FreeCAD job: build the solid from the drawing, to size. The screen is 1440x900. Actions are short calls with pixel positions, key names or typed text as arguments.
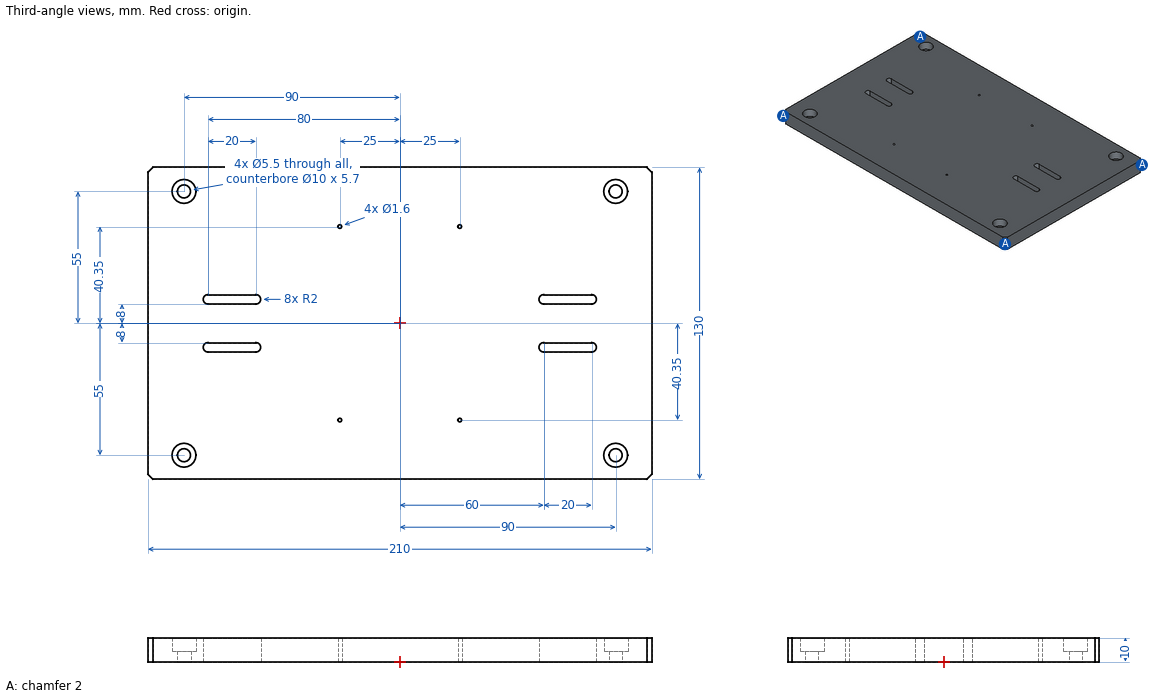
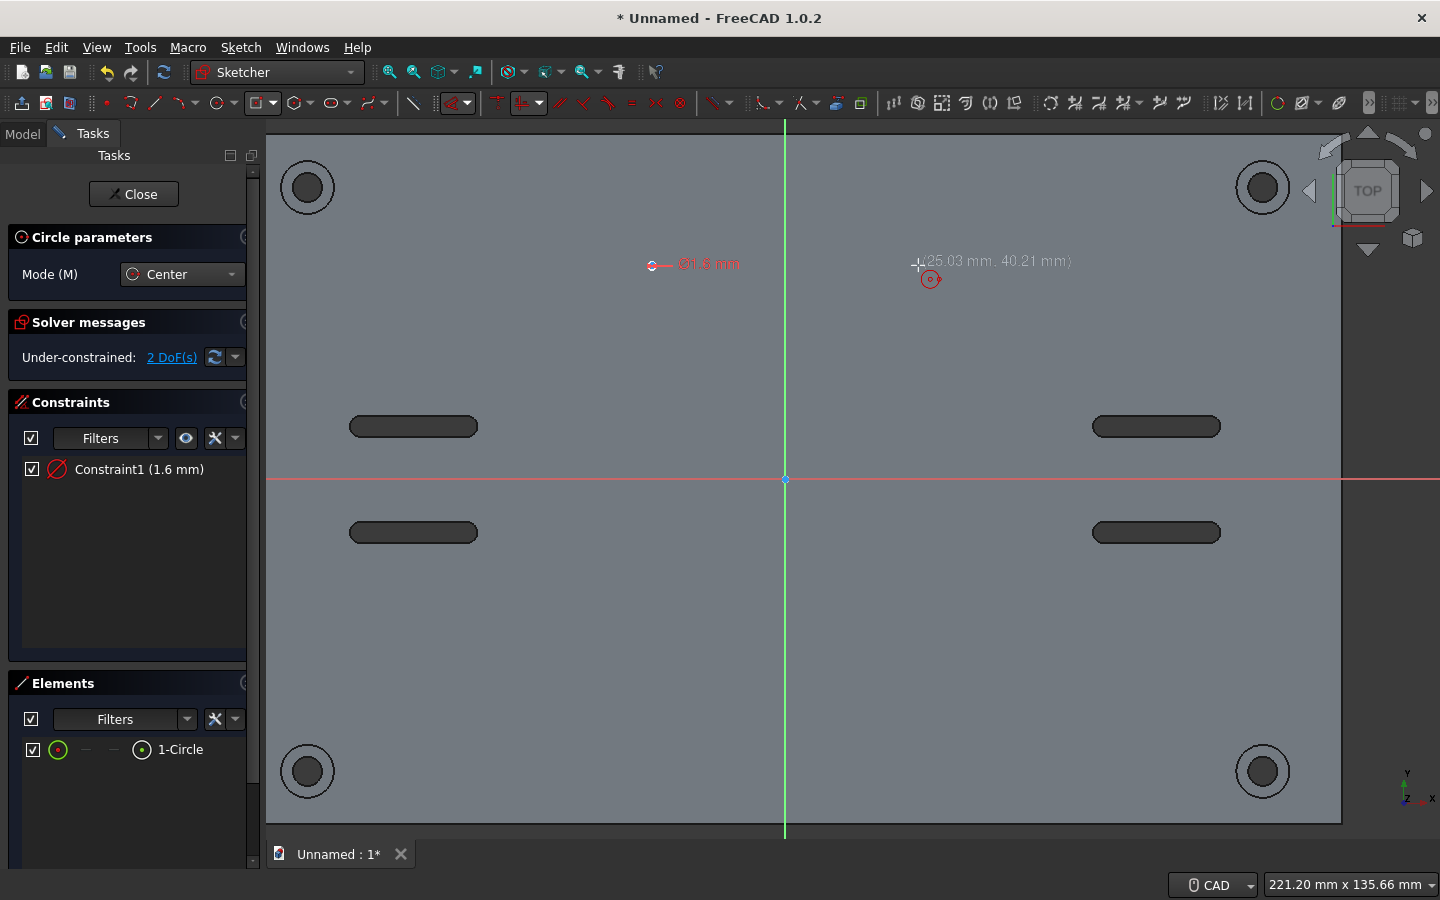
click(918, 265)
move(921, 262)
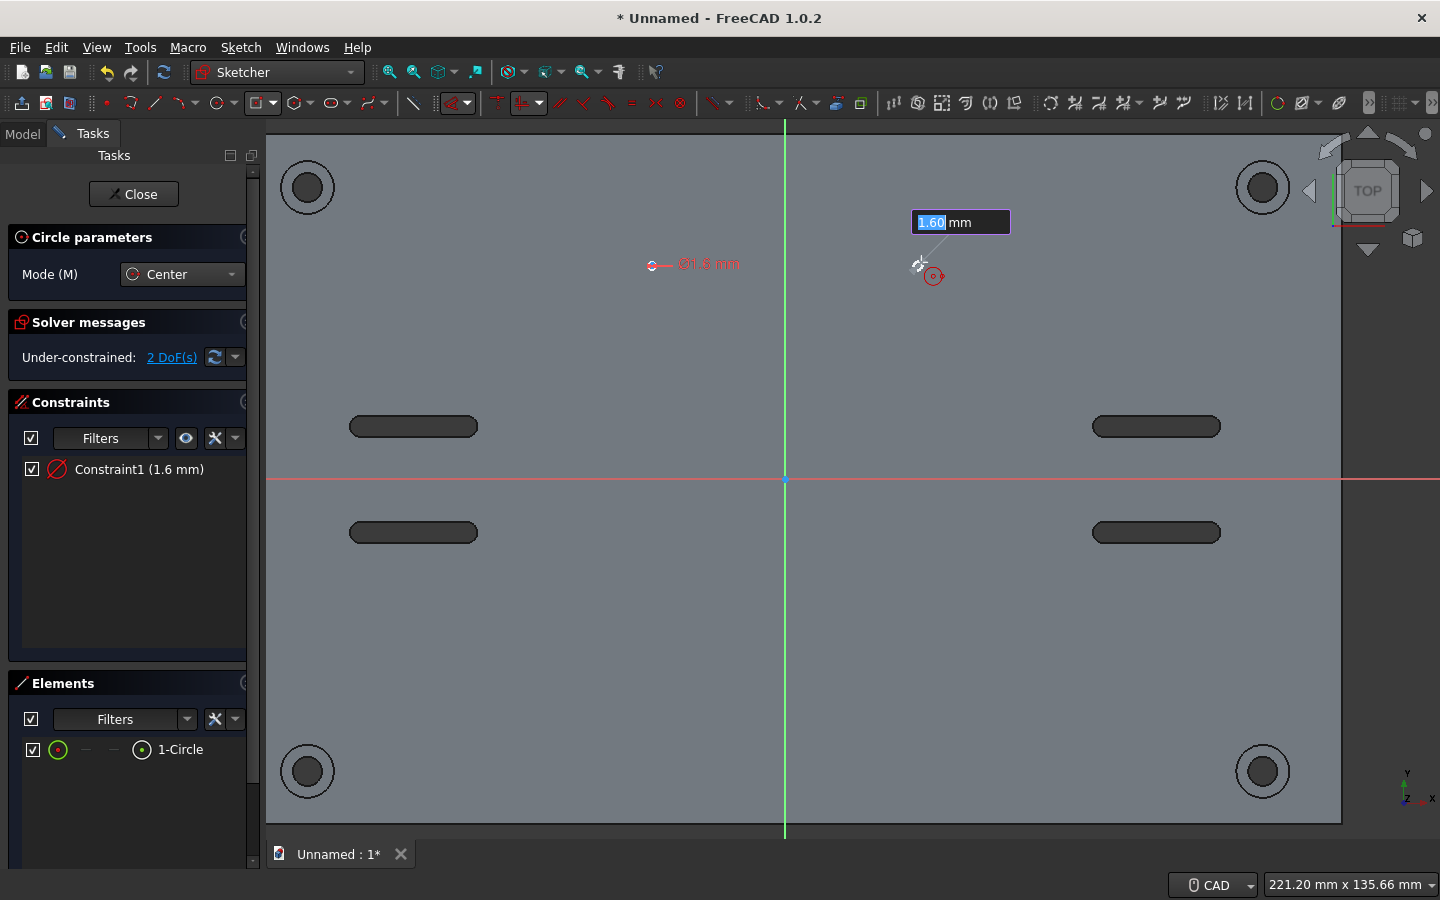
text(1.6)
key(Return)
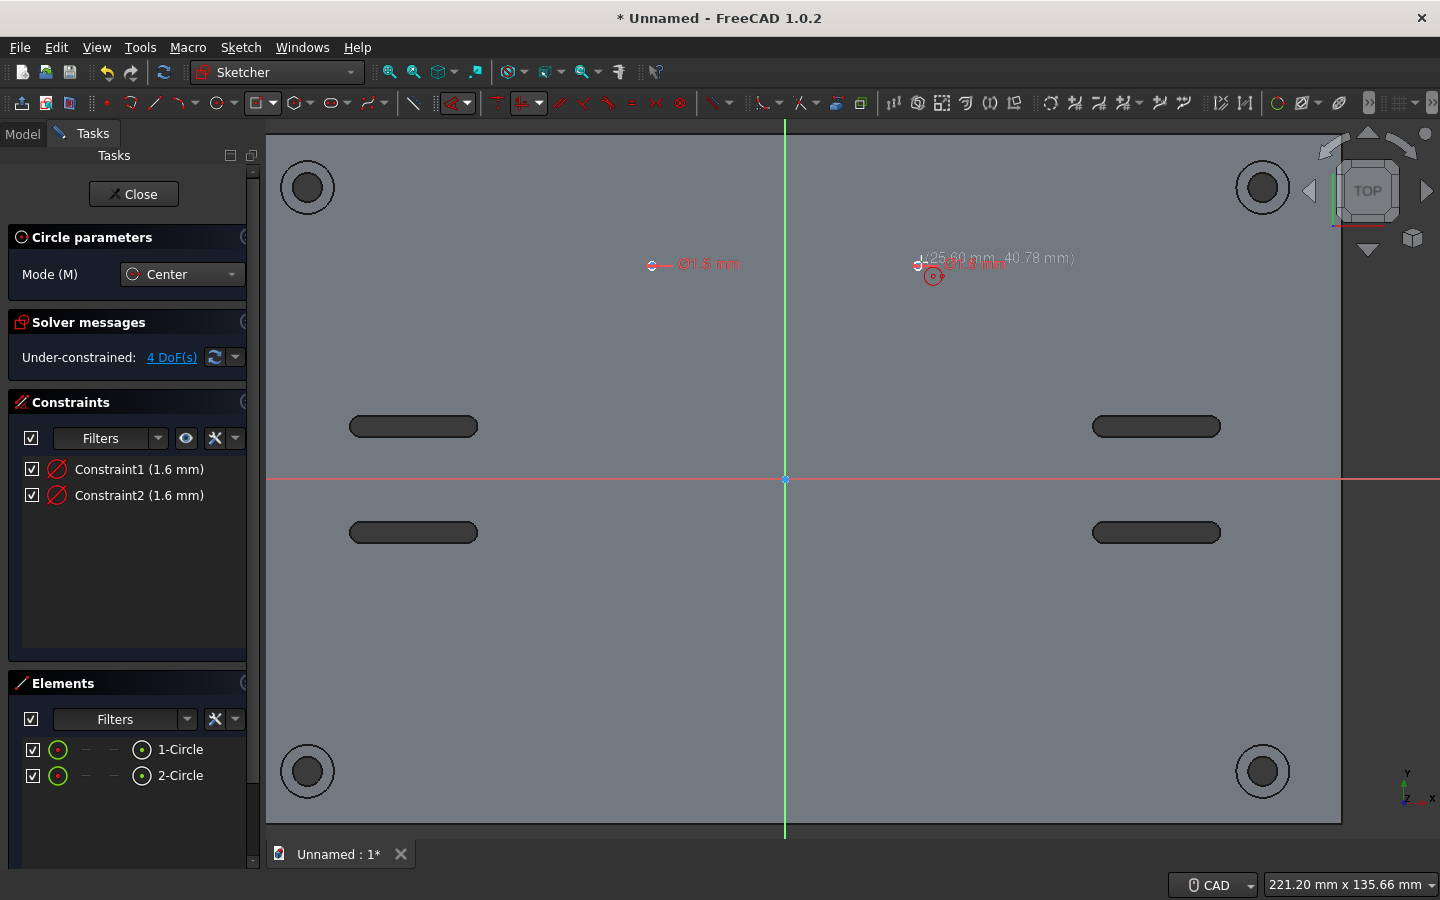
scroll(918, 694, up, 9)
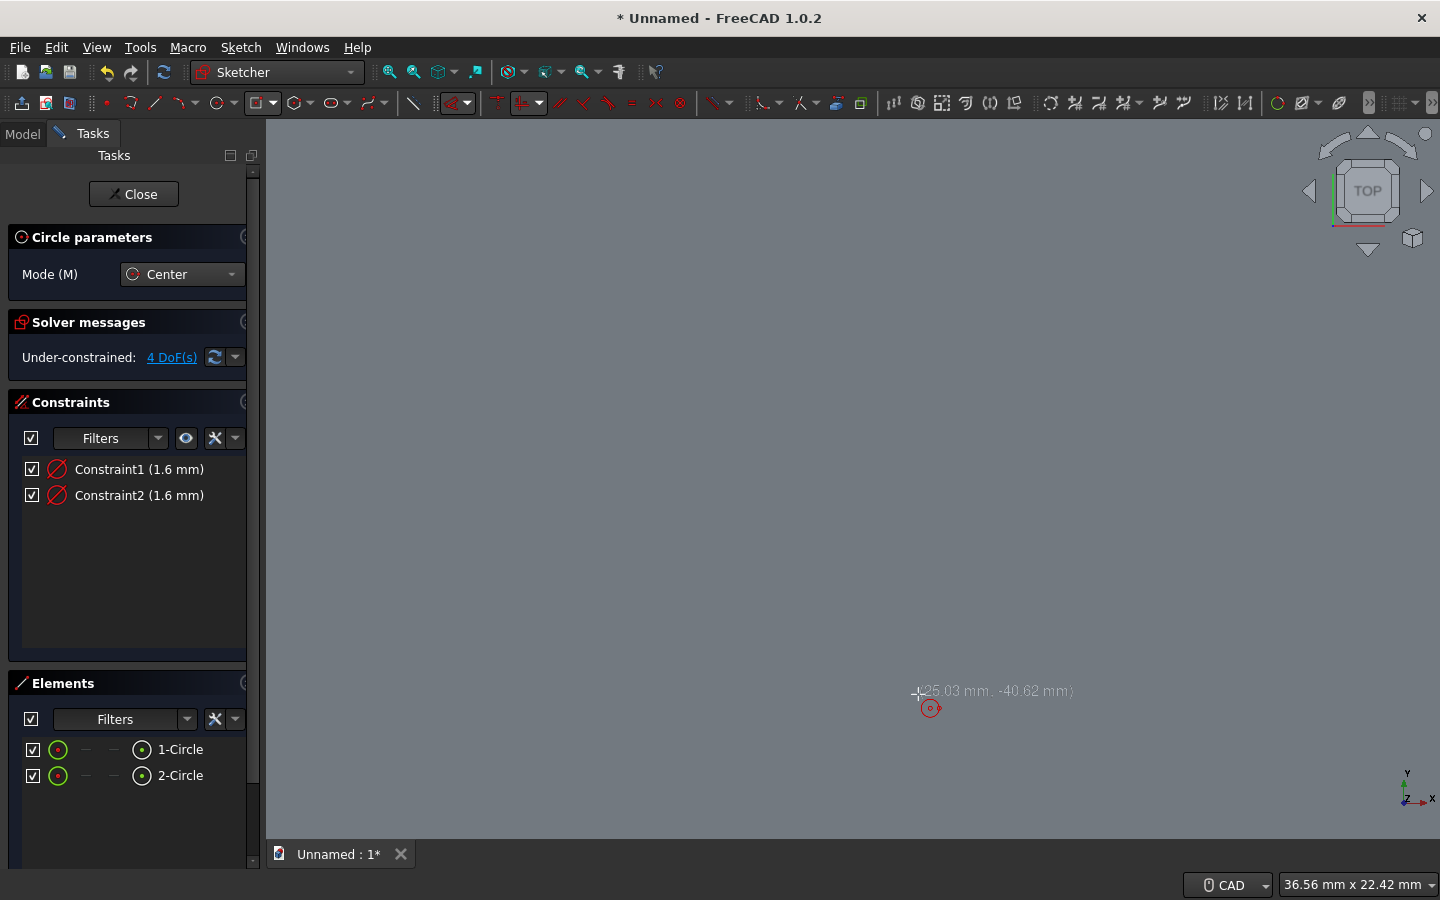
scroll(918, 694, down, 9)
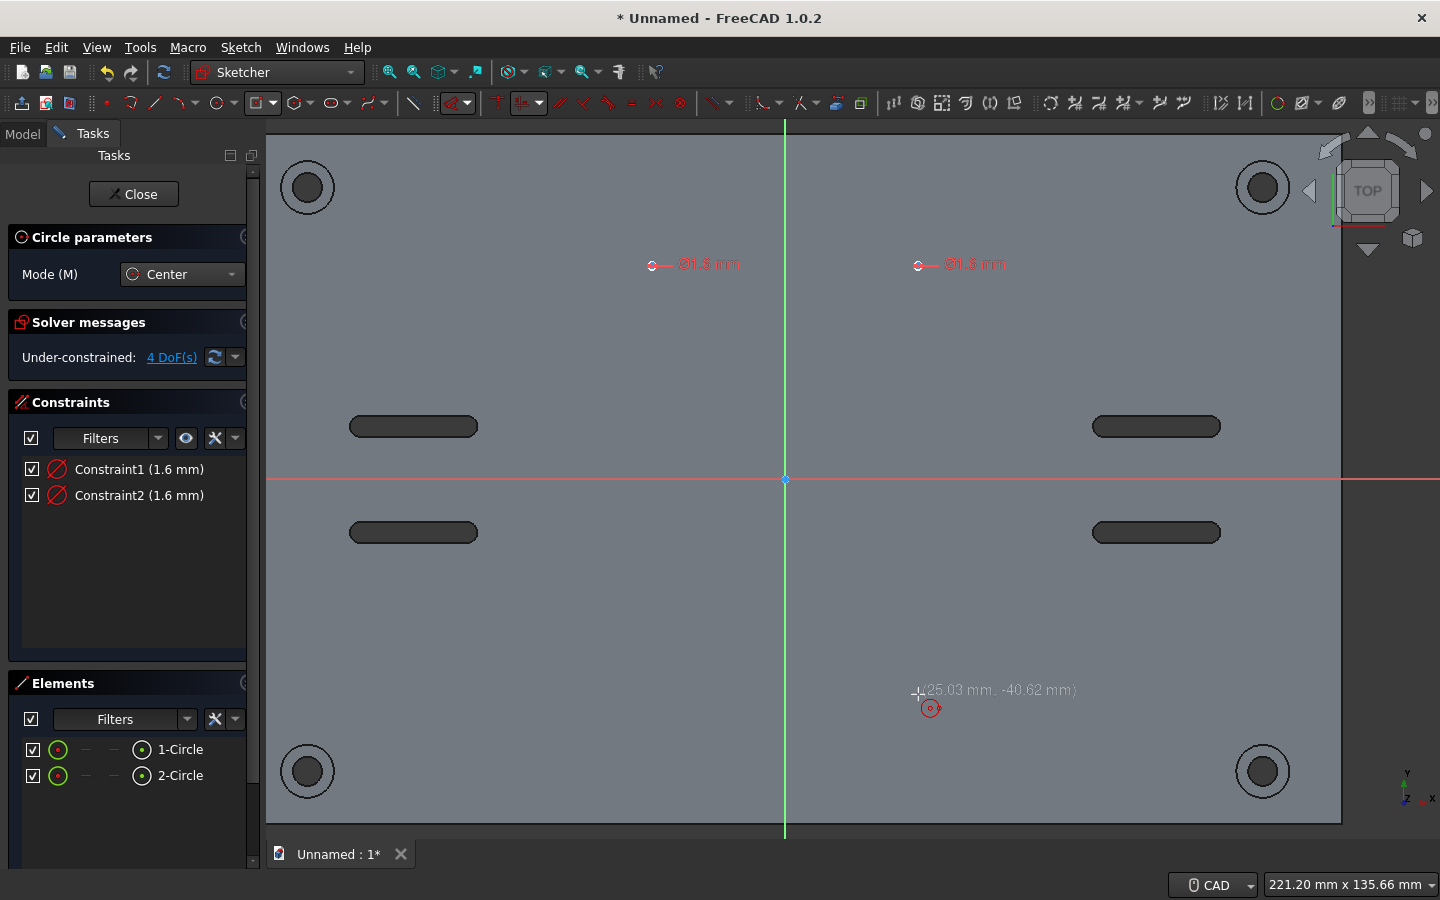
click(918, 694)
move(921, 691)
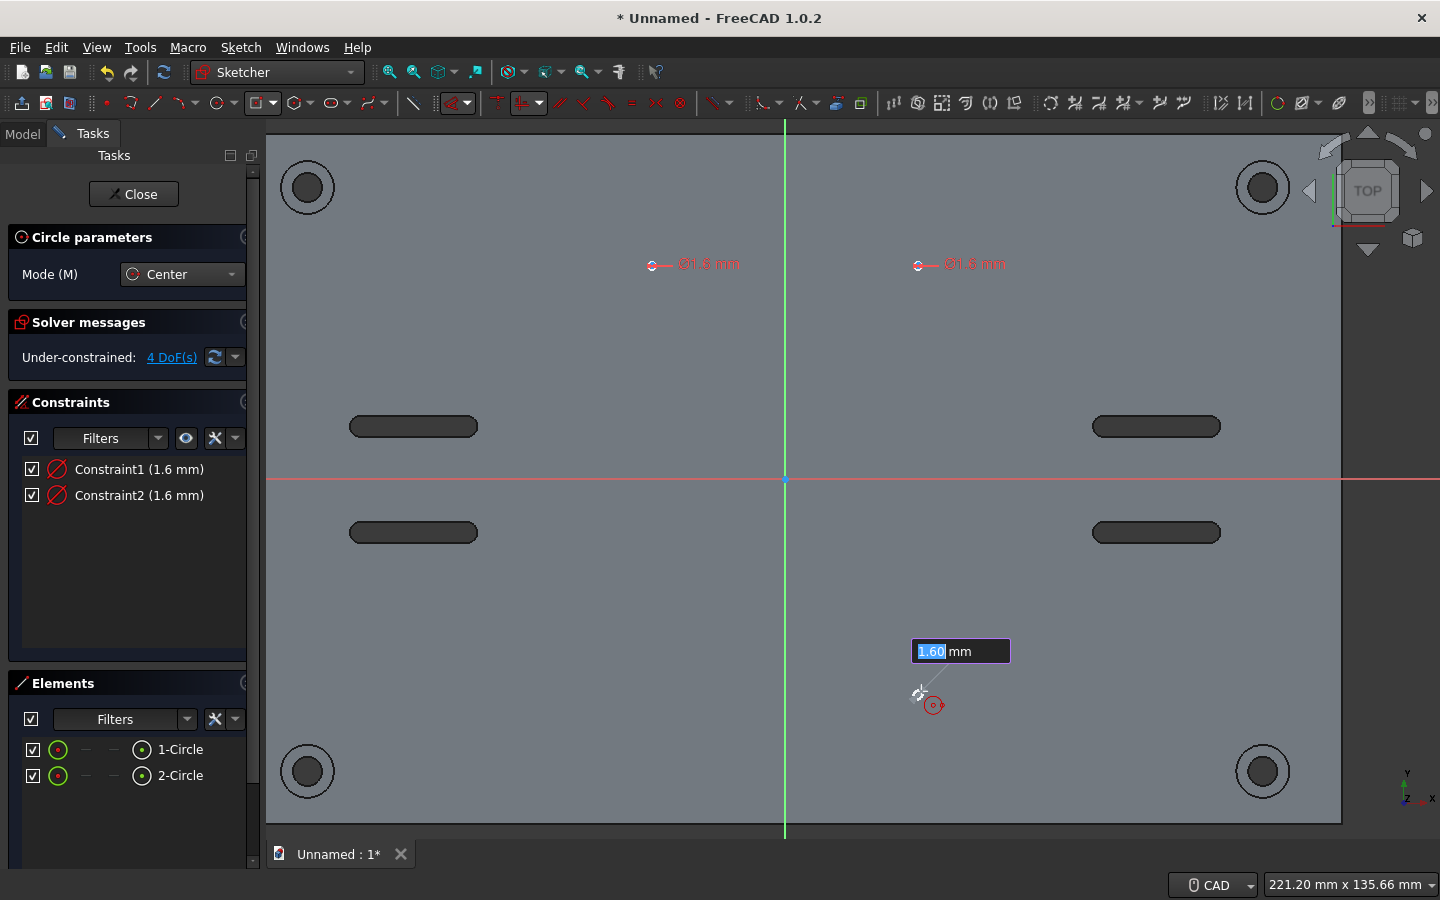
text(1.6)
key(Return)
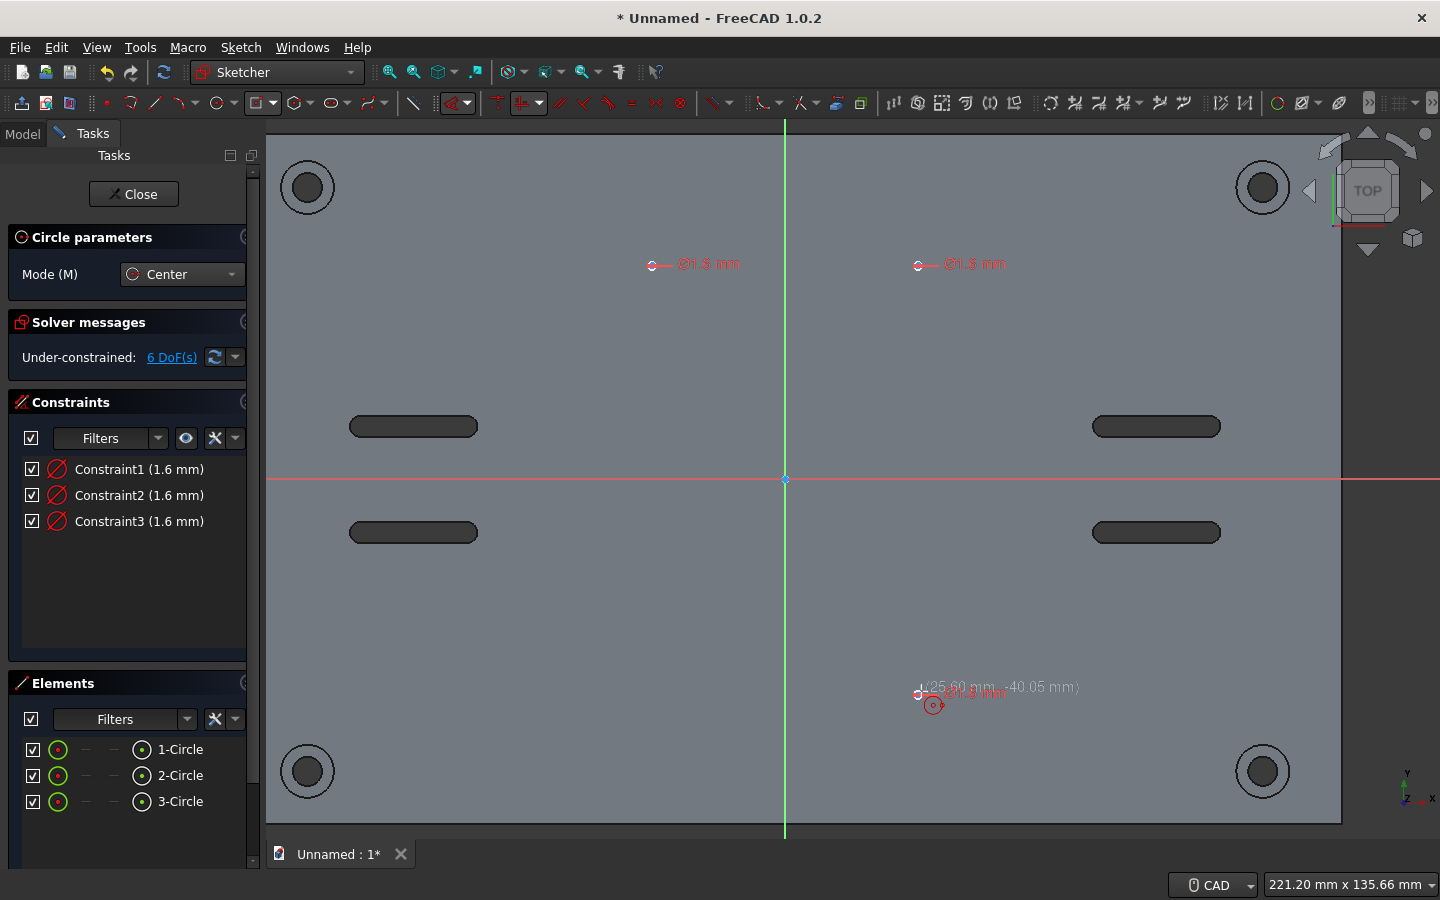
scroll(652, 694, up, 9)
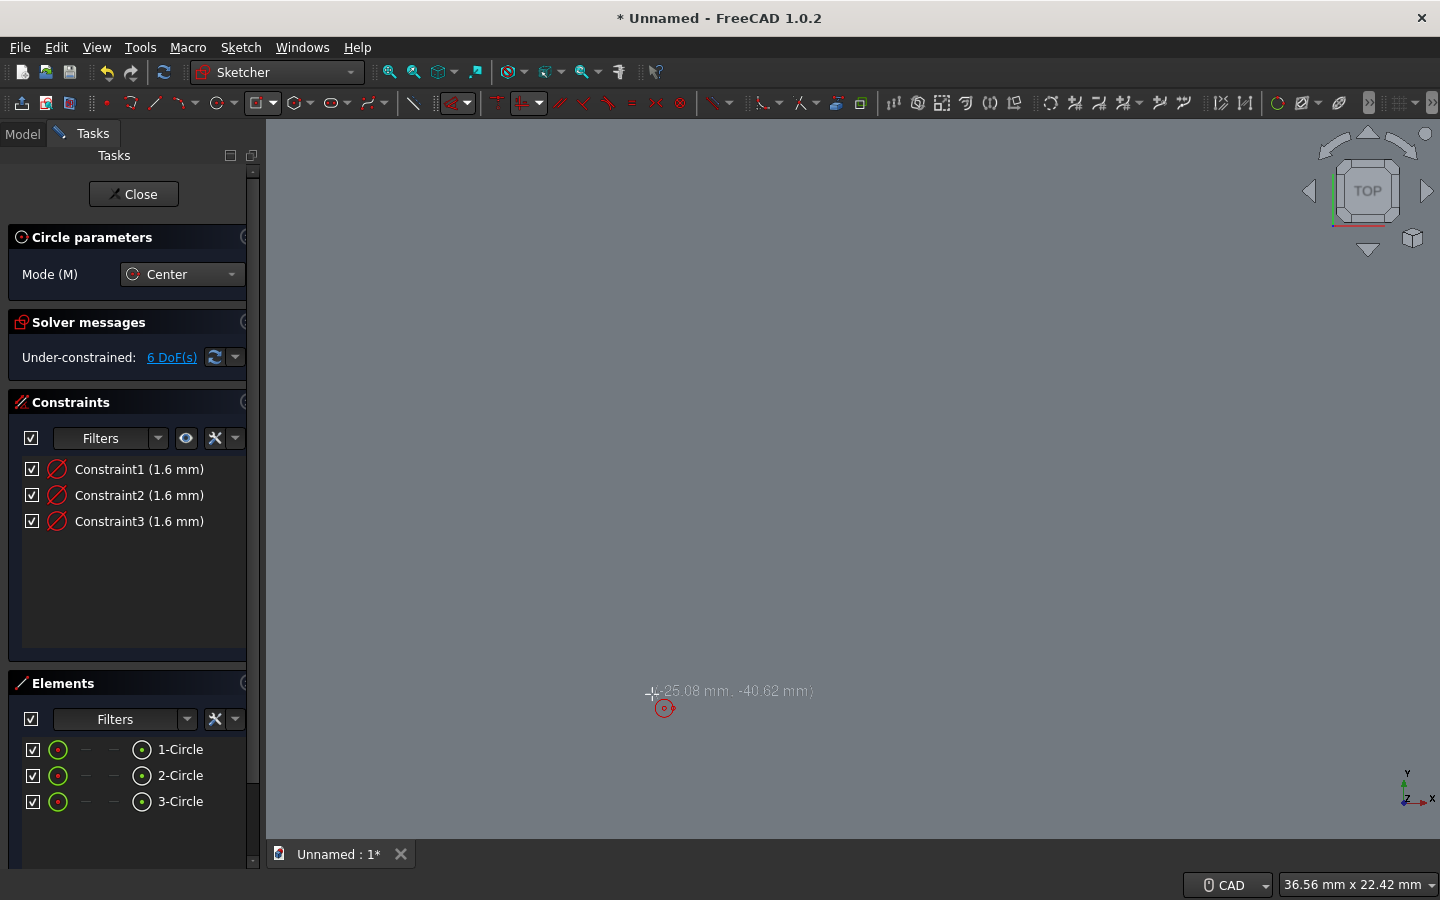
scroll(652, 694, down, 9)